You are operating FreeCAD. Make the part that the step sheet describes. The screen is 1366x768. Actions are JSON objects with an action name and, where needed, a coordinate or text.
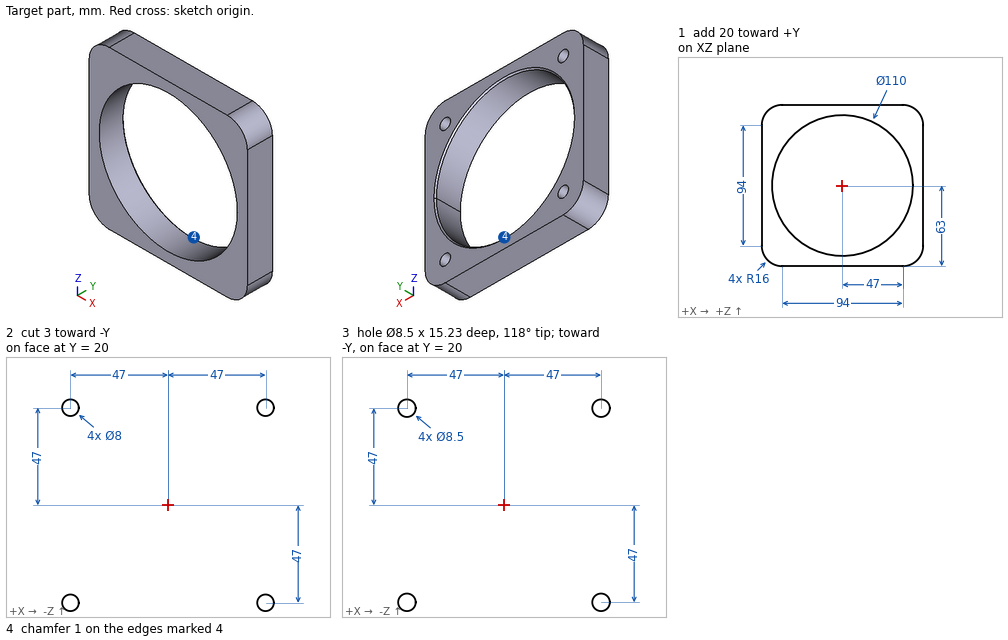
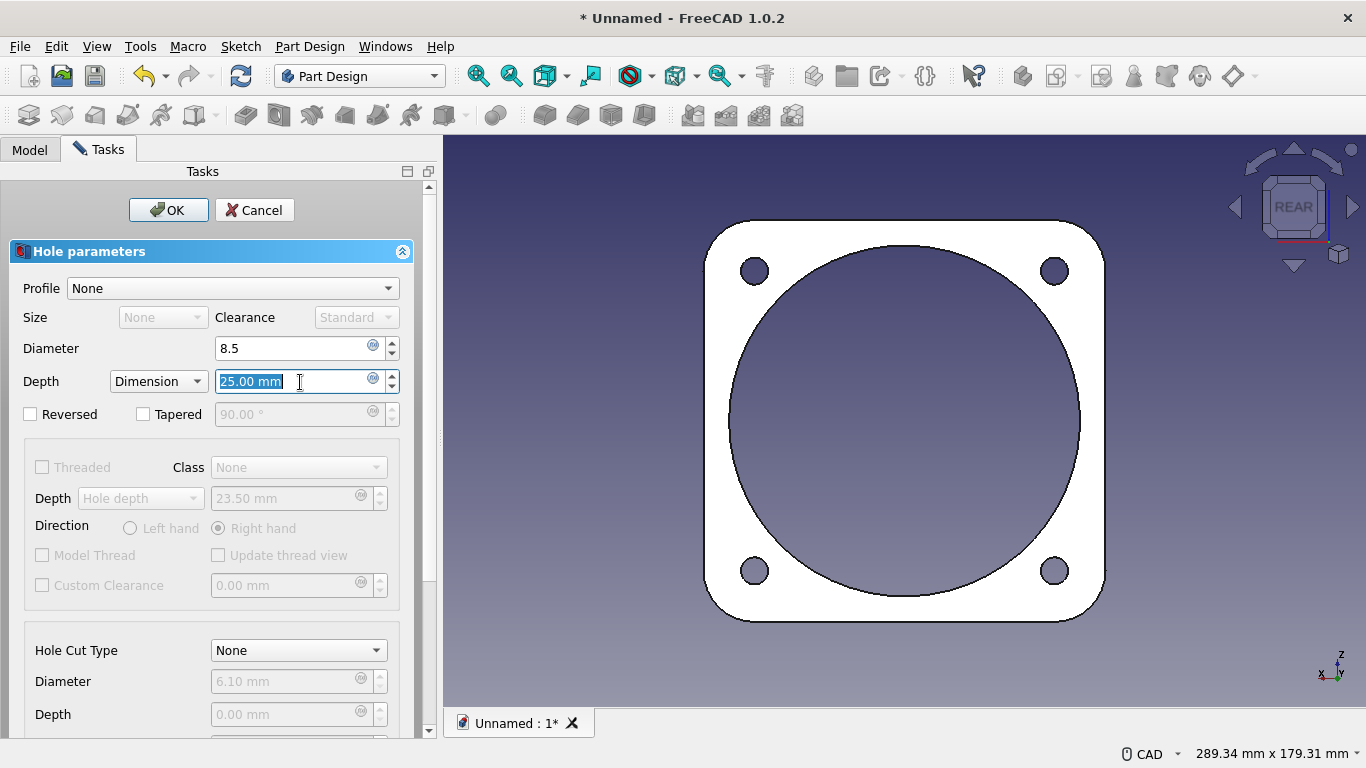
{"action": "type", "text": "15.23"}
{"action": "key", "text": "Tab"}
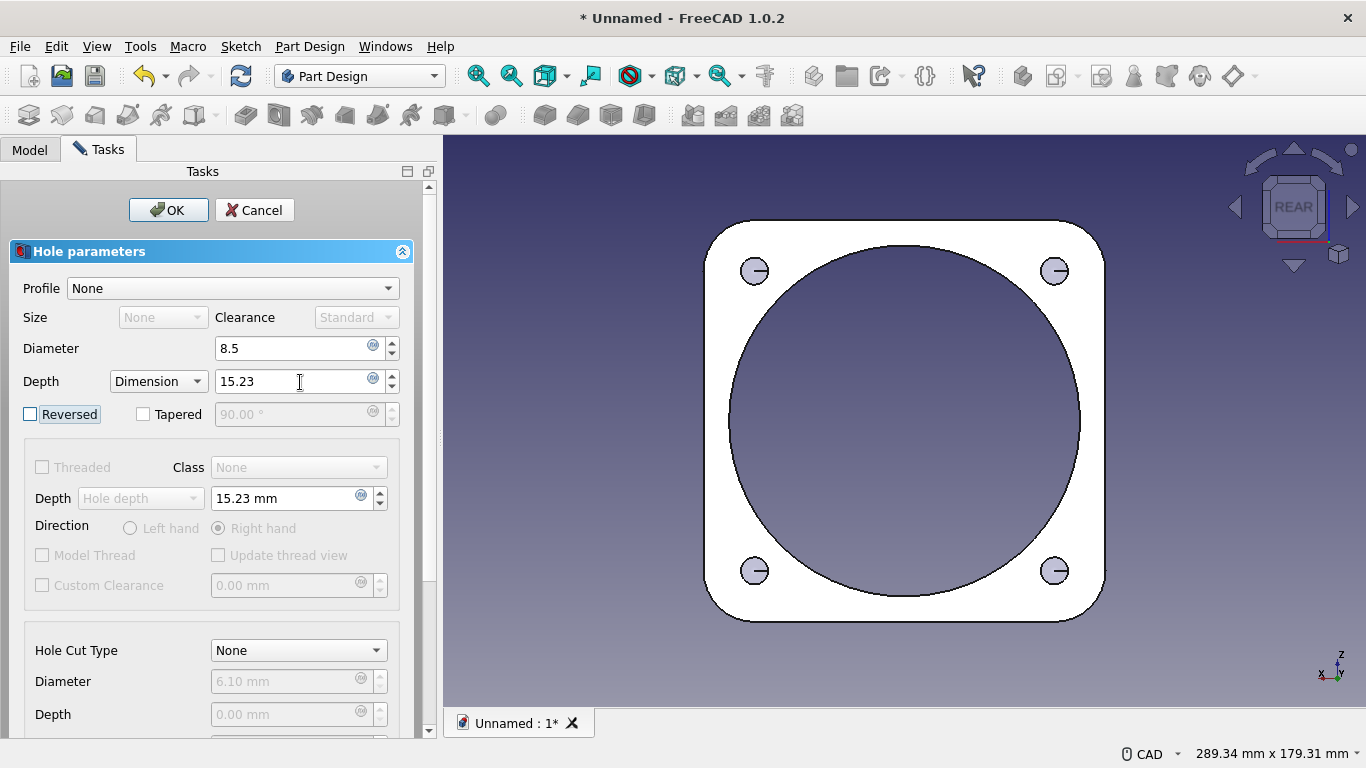
{"action": "left_click", "coordinate": [169, 210]}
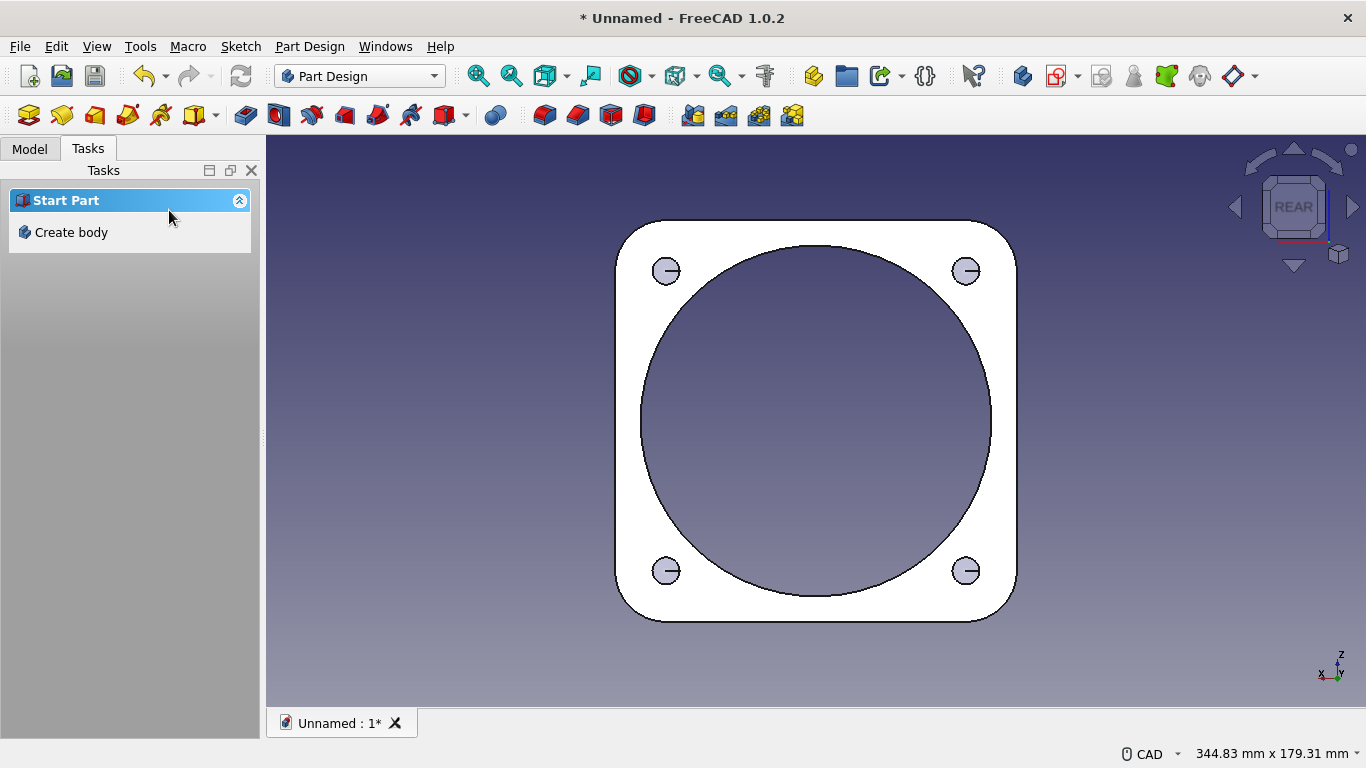
{"action": "left_click", "coordinate": [958, 317]}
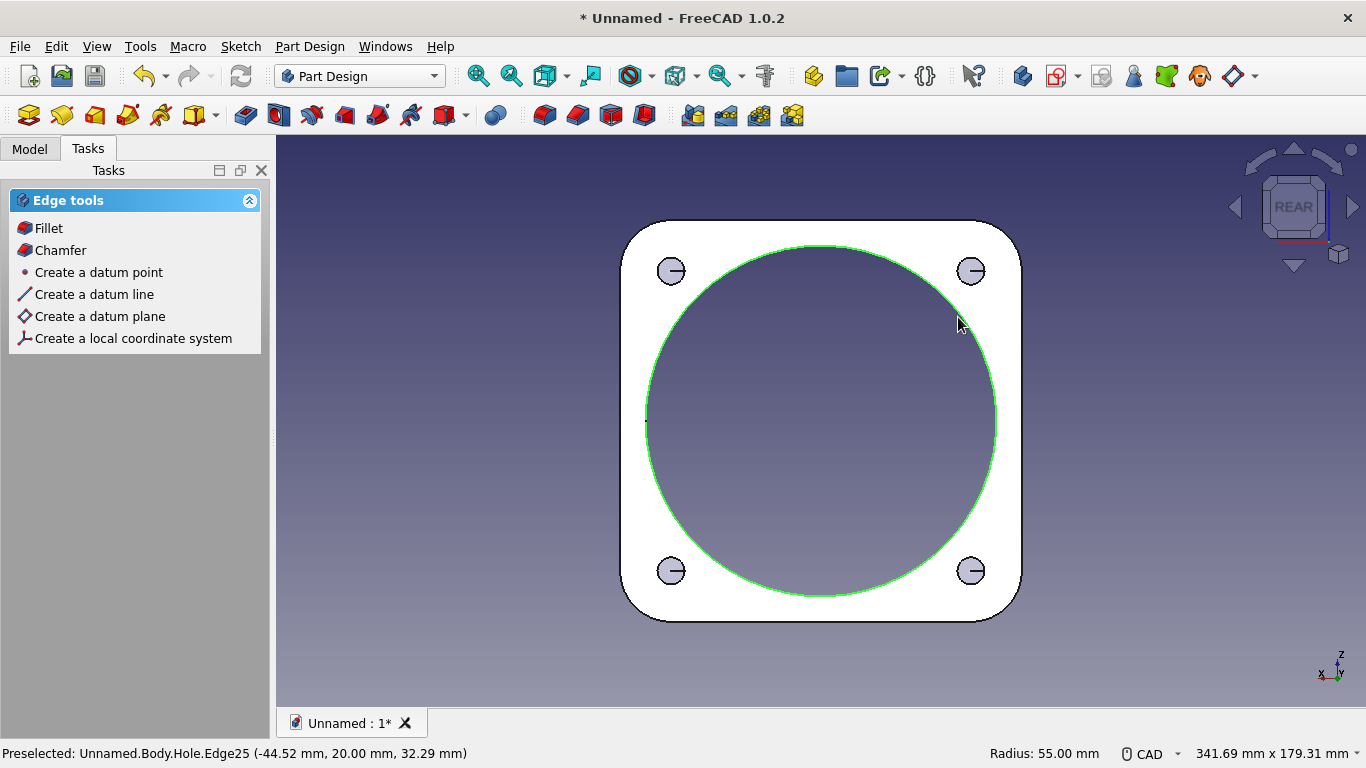
{"action": "left_click", "coordinate": [578, 116]}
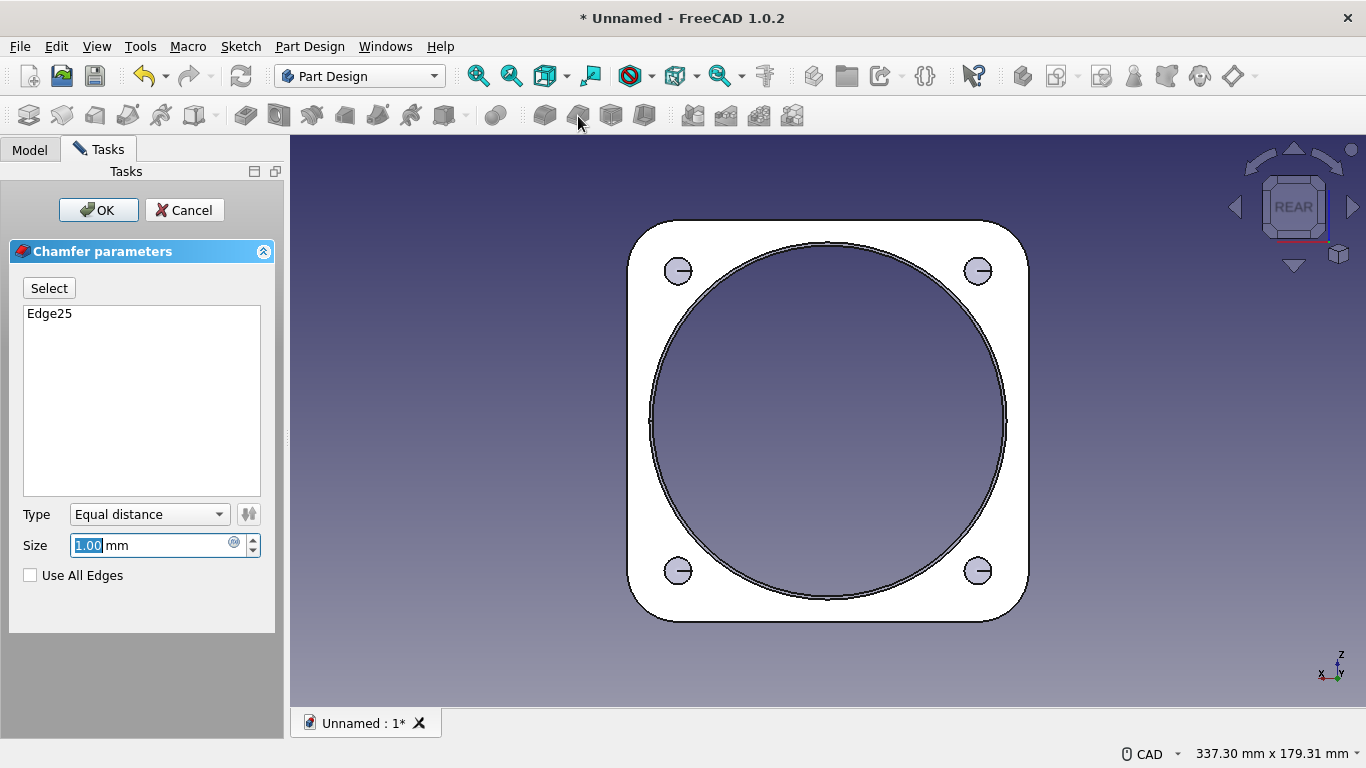
{"action": "type", "text": "1"}
{"action": "key", "text": "Tab"}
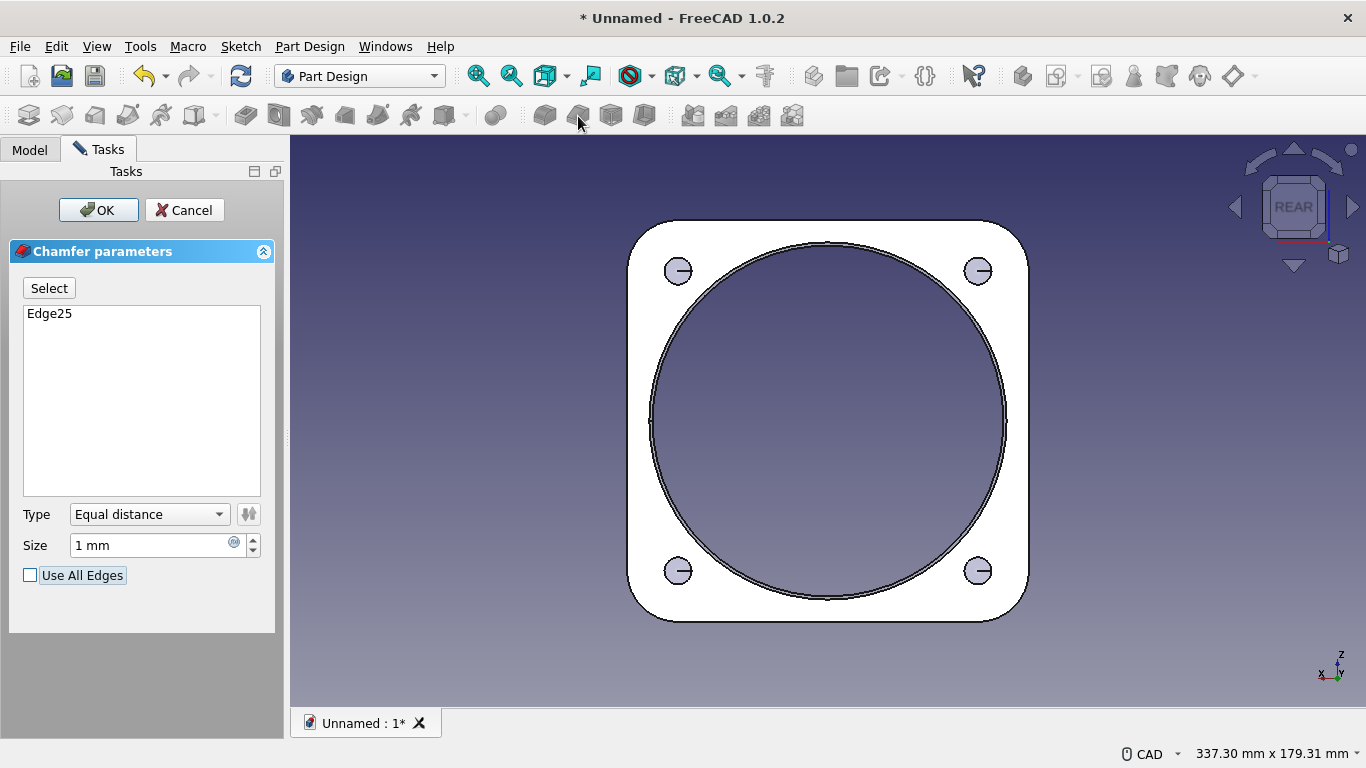
{"action": "left_click", "coordinate": [99, 210]}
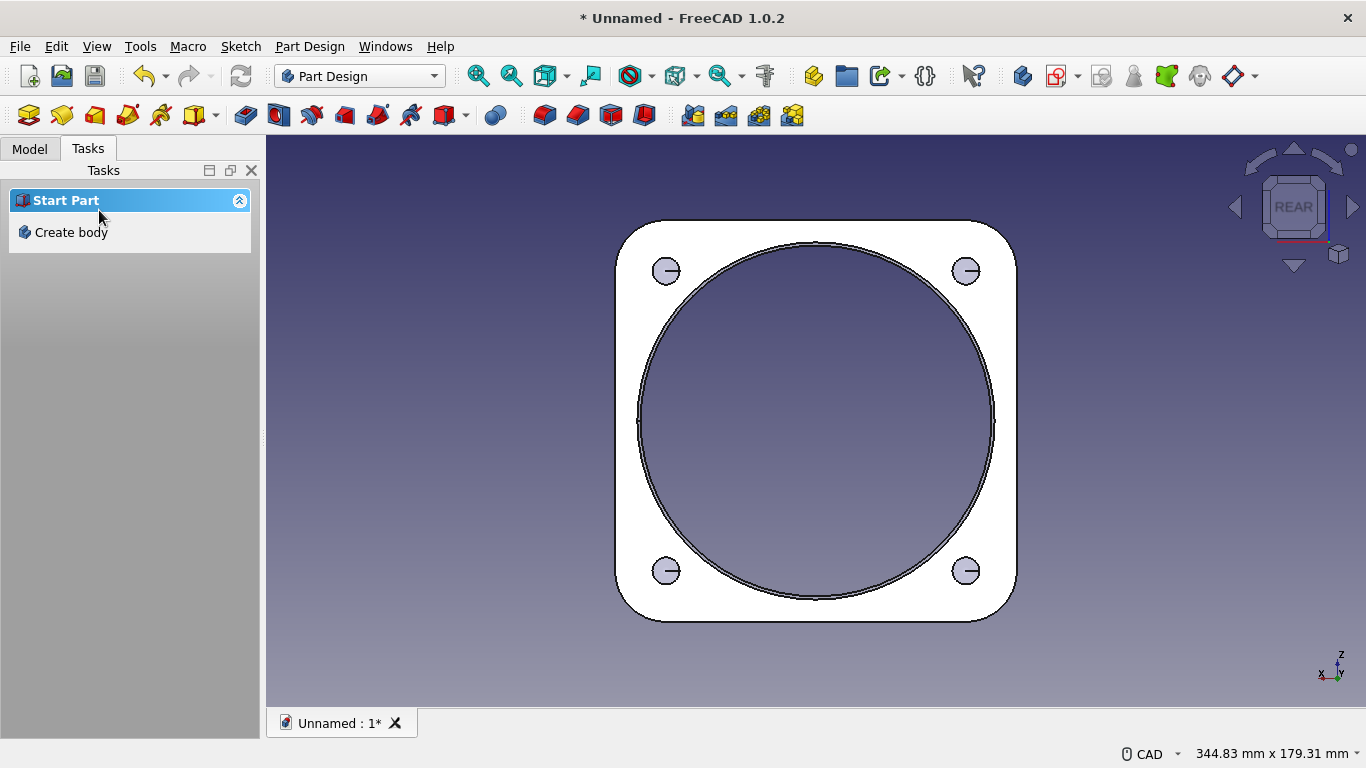
{"action": "key", "text": "0"}